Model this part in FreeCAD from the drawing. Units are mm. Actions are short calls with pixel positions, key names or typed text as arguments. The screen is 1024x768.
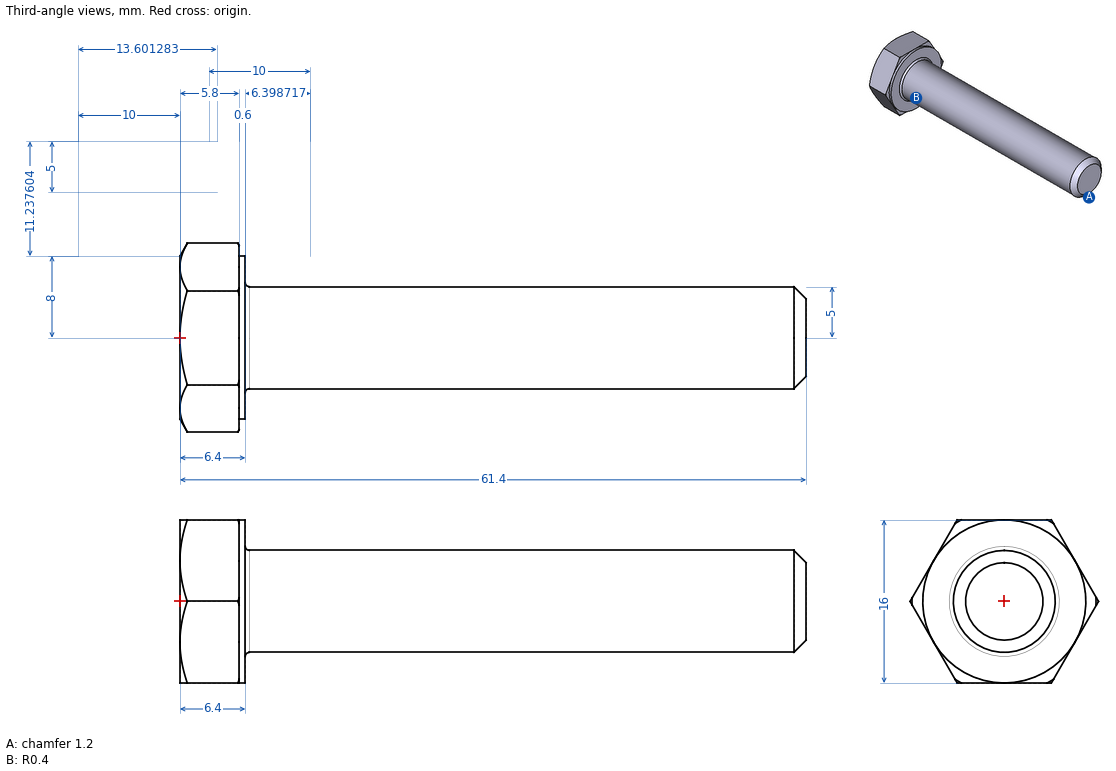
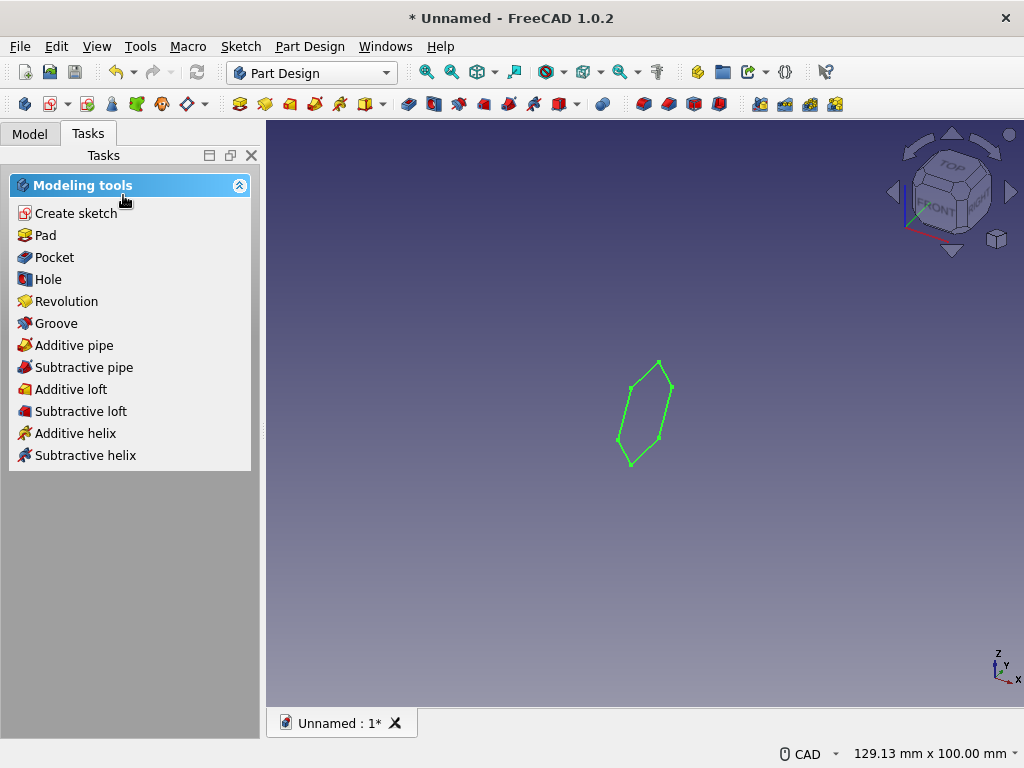
click(240, 104)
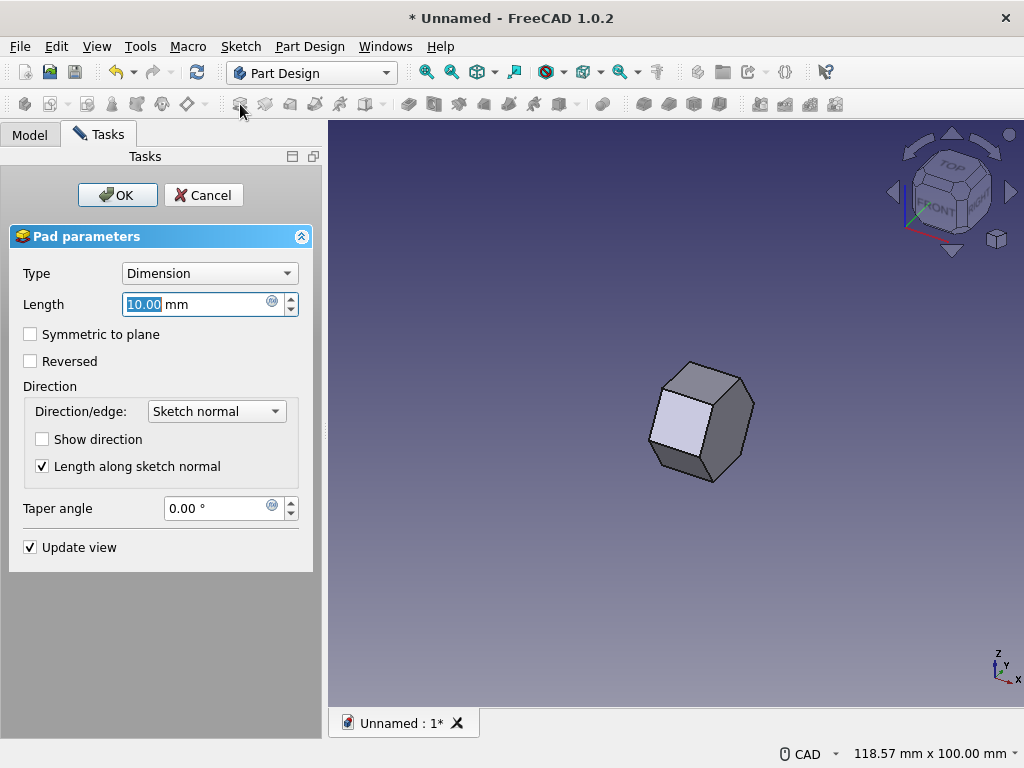
text(6.4)
key(Tab)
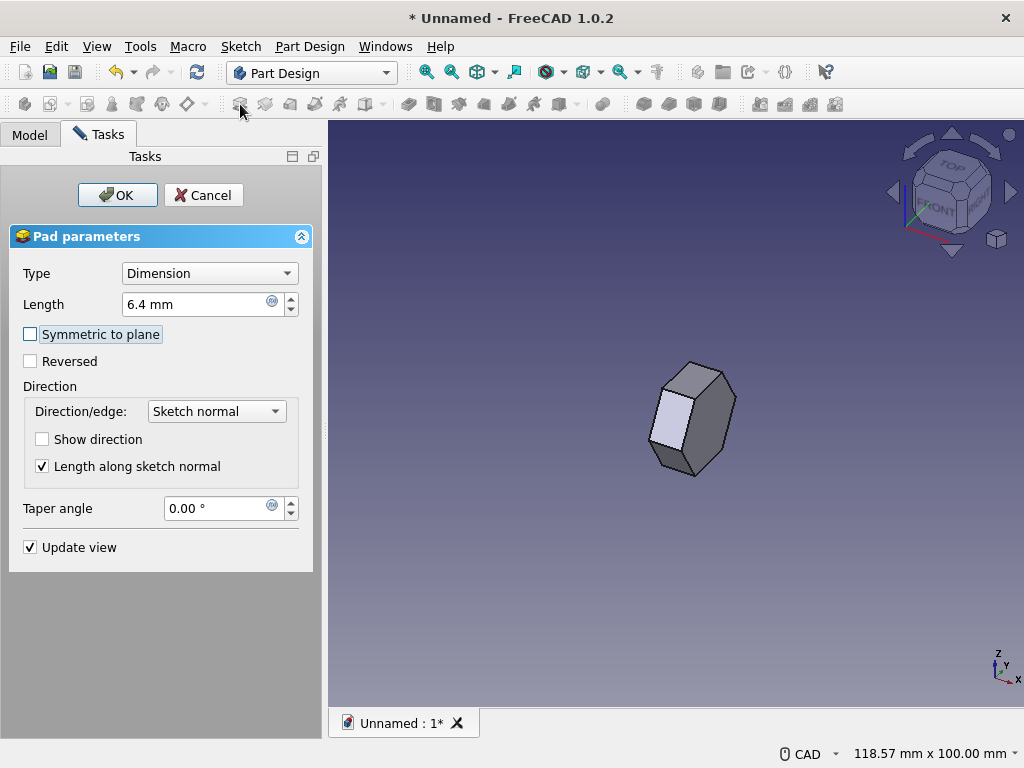
click(118, 195)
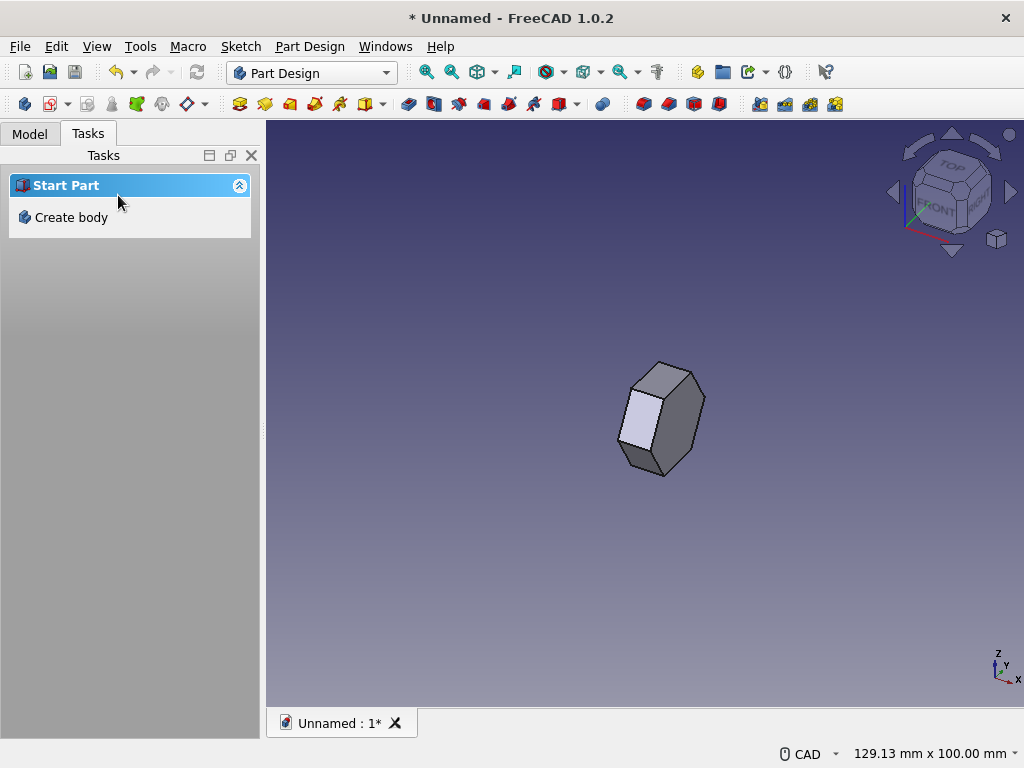
click(427, 72)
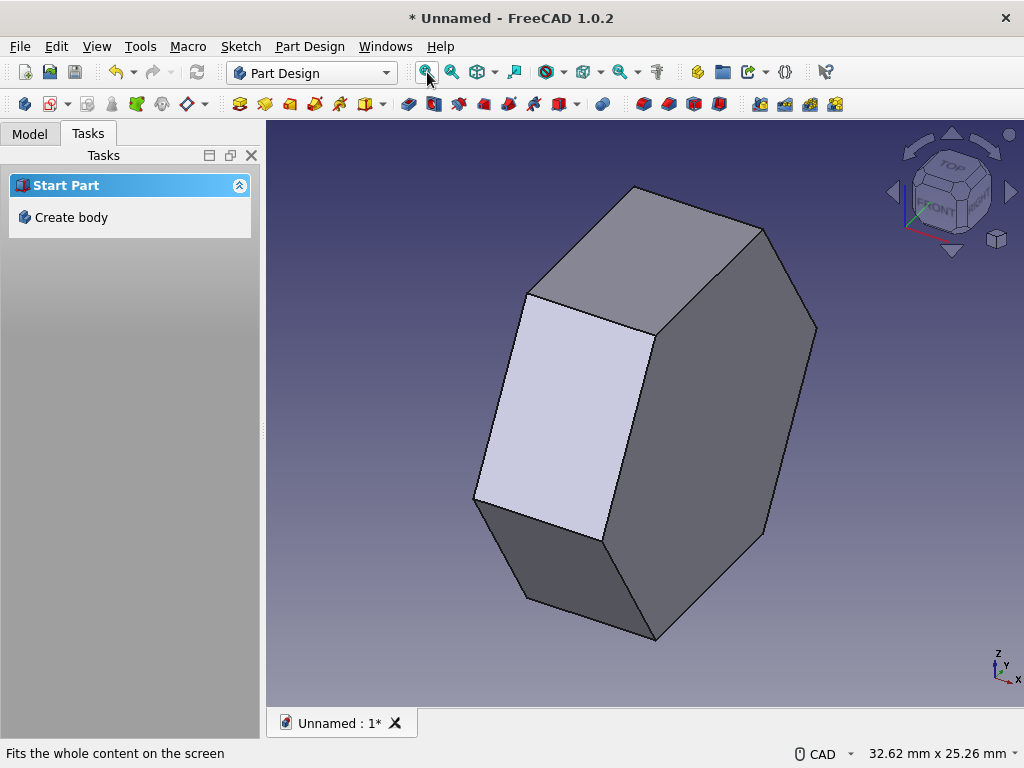
click(50, 104)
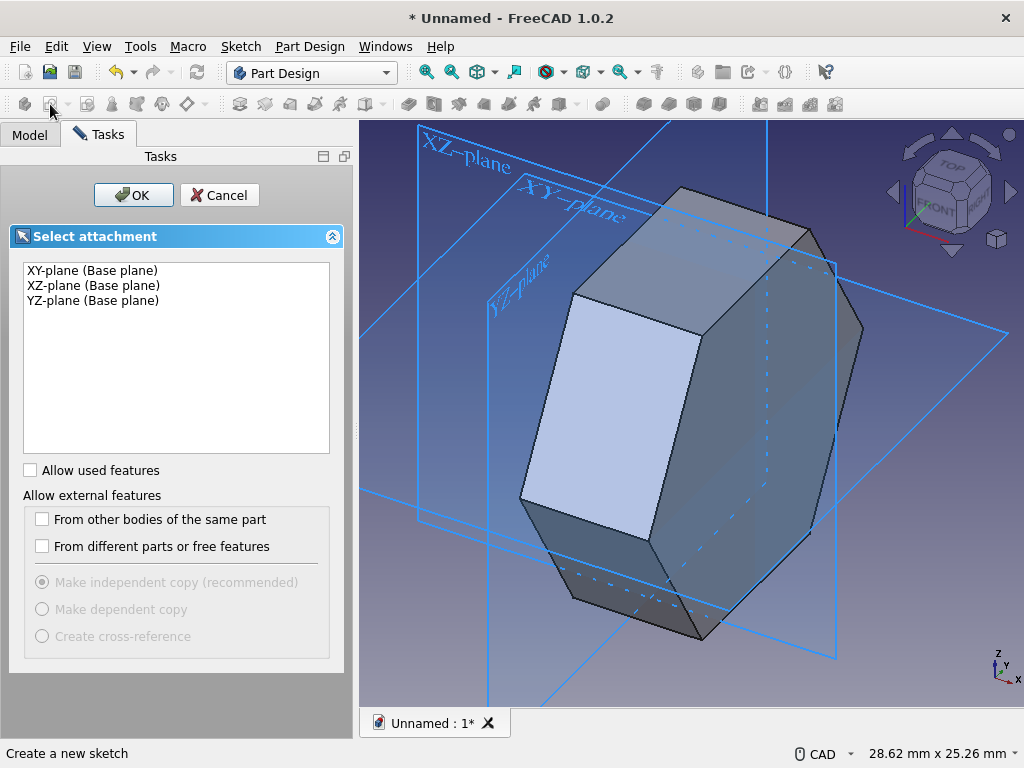
click(84, 270)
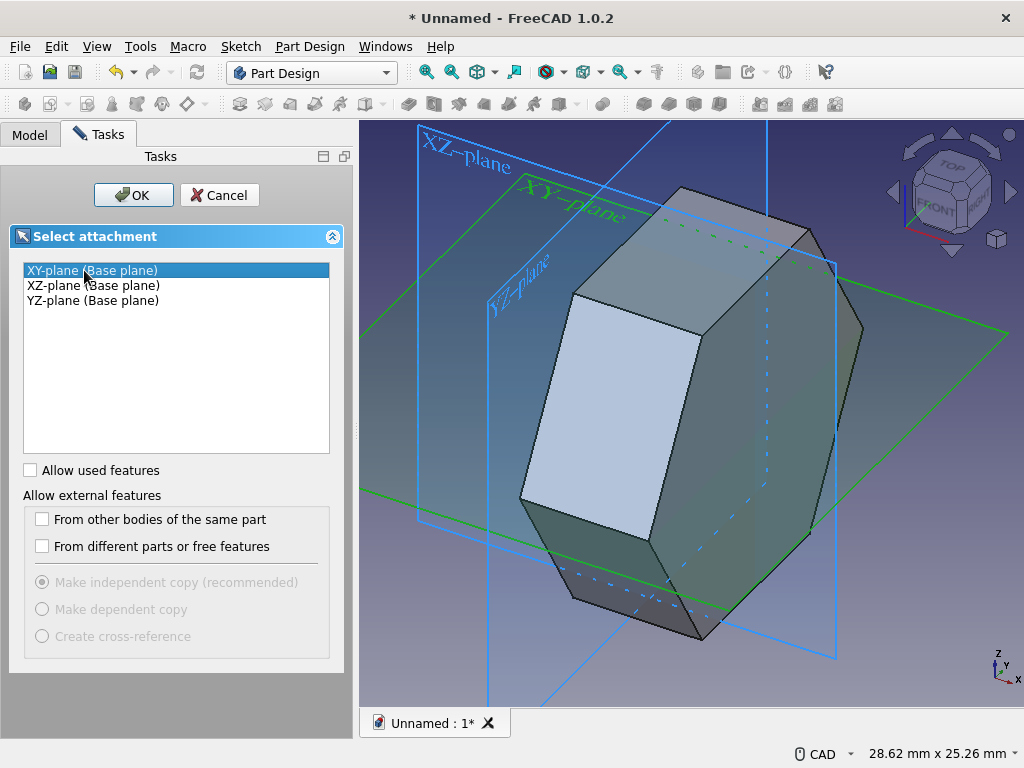
click(134, 195)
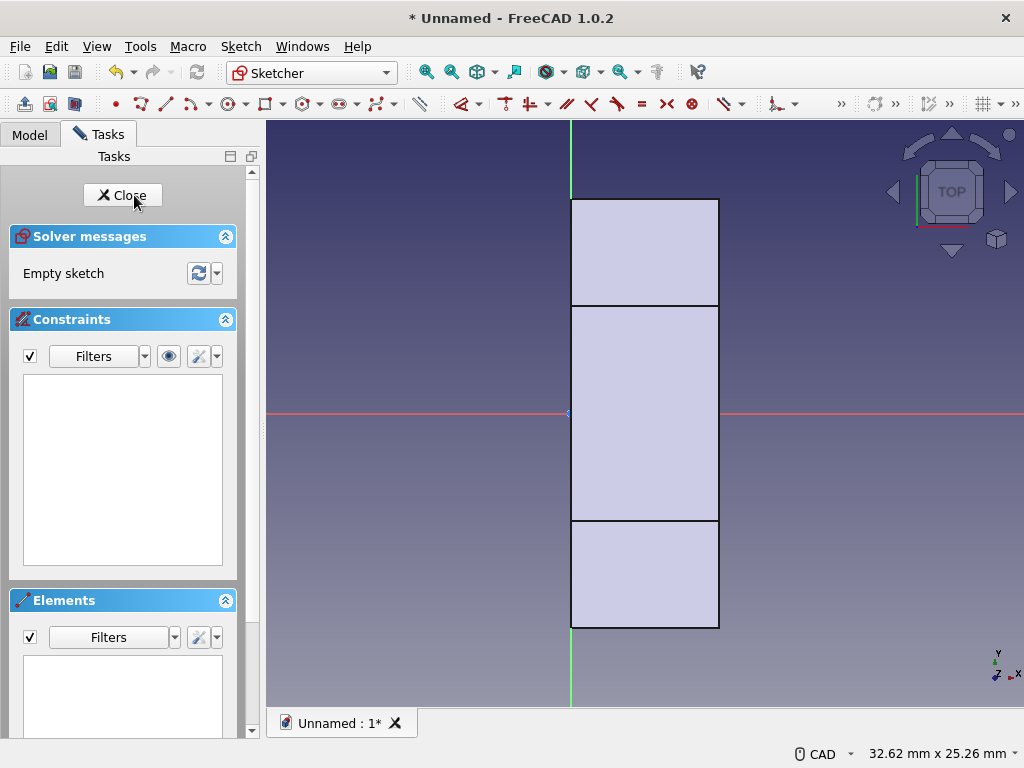
click(75, 104)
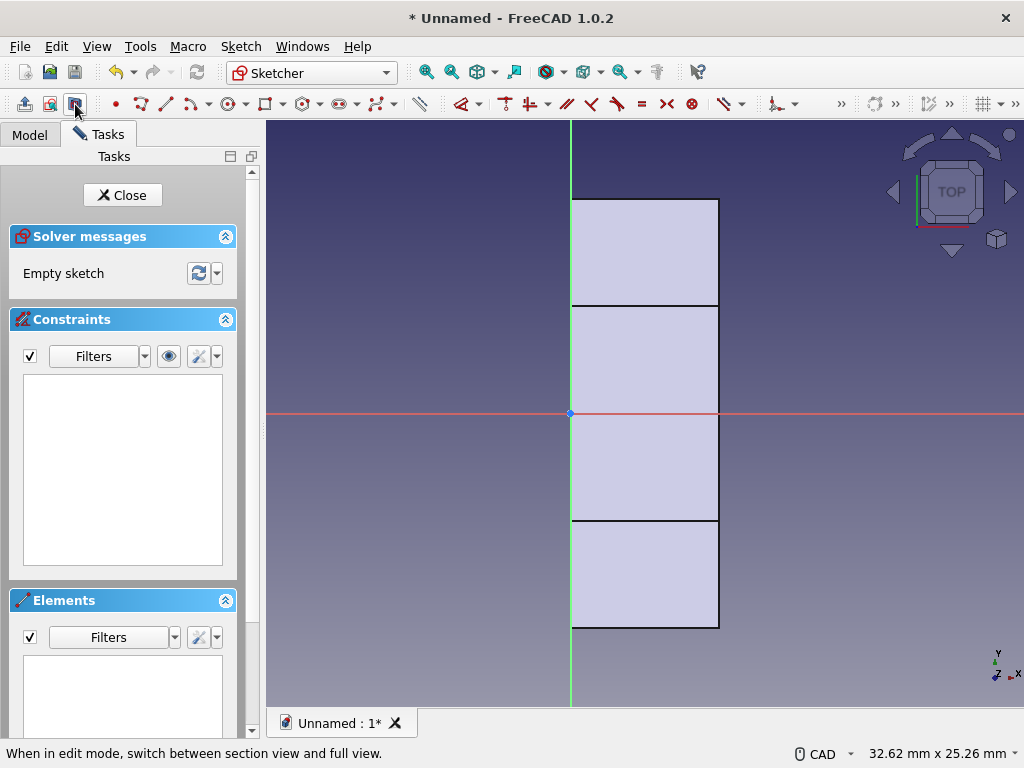
scroll(294, 439, down, 6)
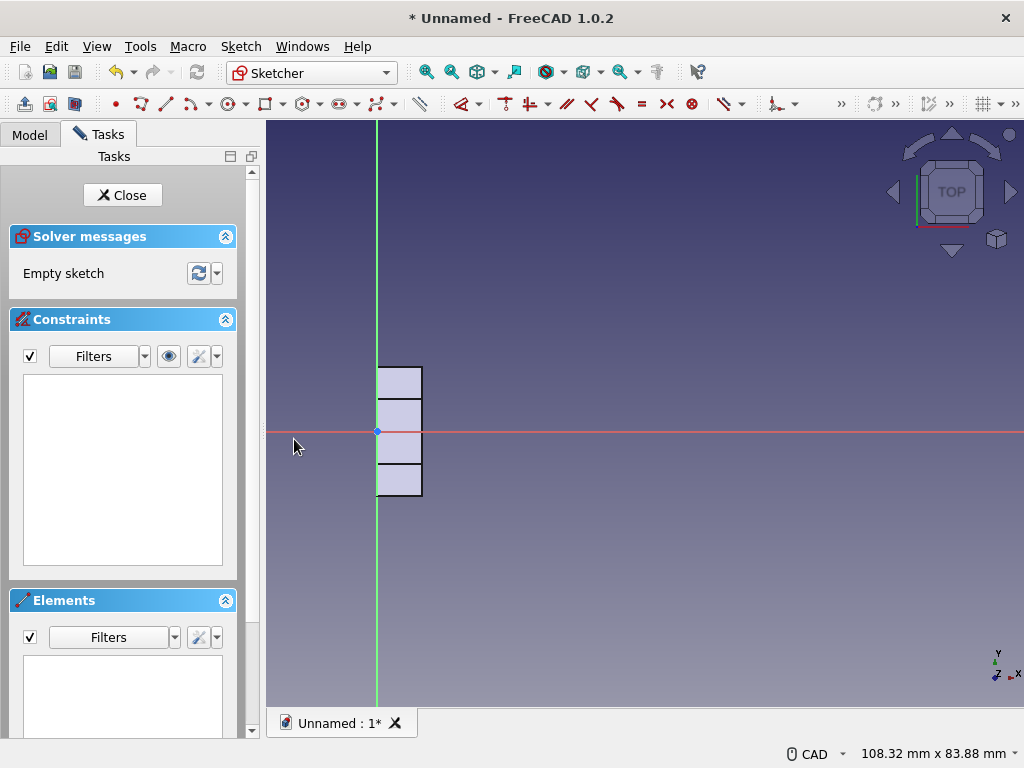
click(264, 104)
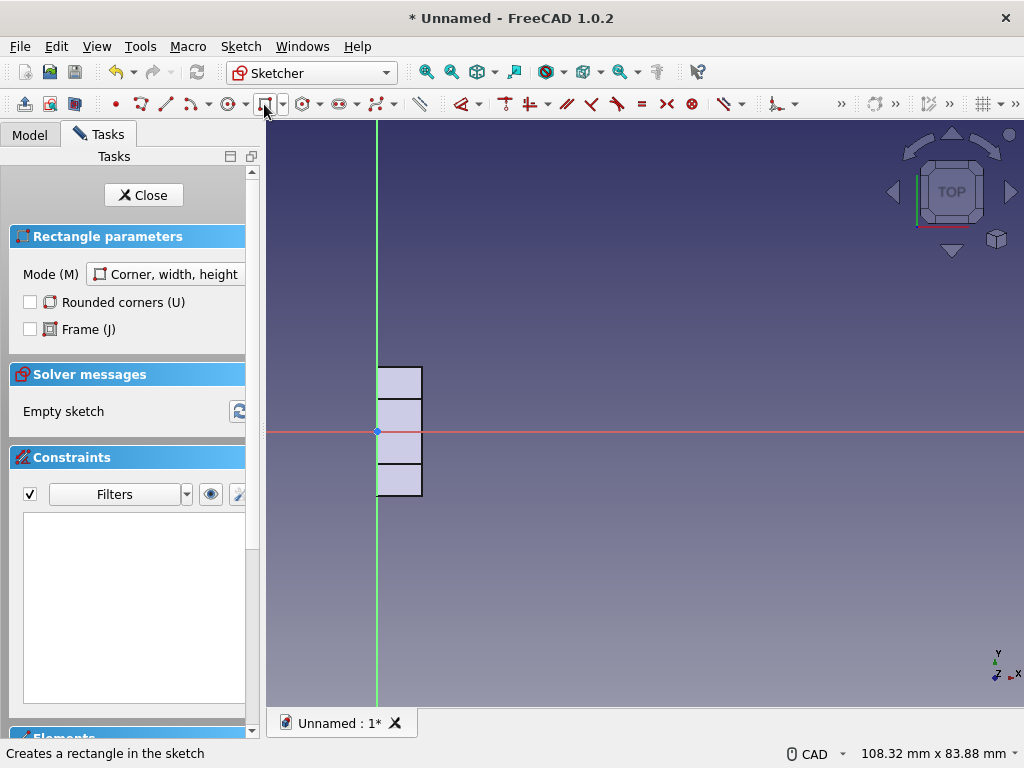
click(377, 432)
move(807, 397)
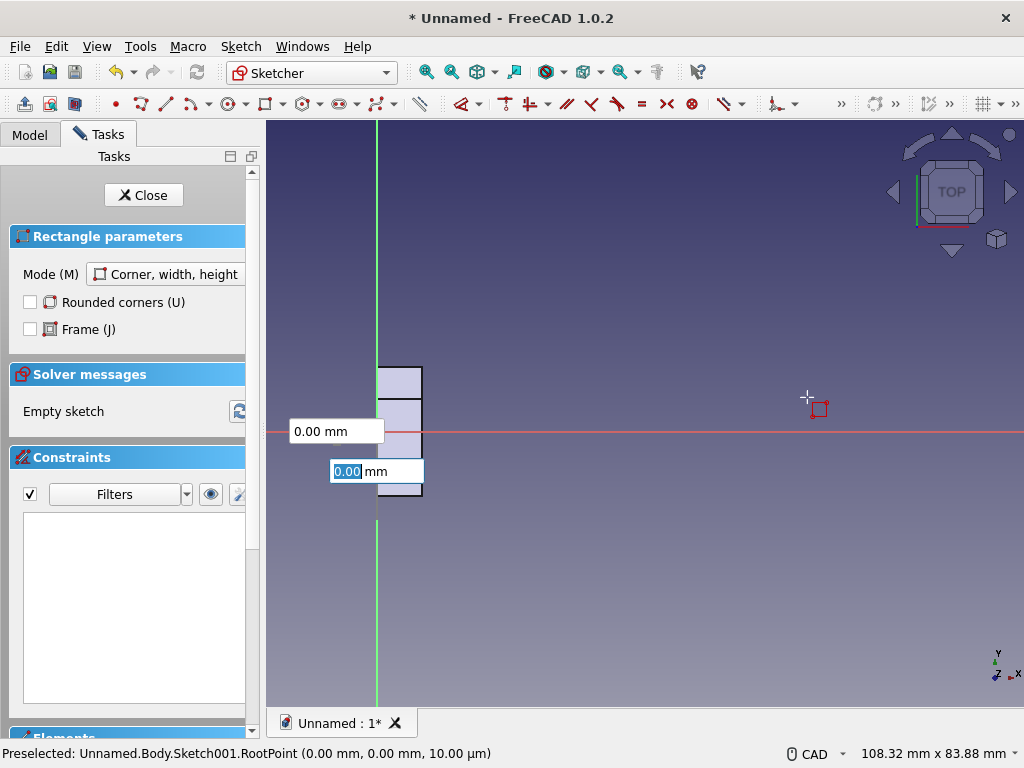
text(61.4)
key(Tab)
text(5)
key(Return)
key(Escape)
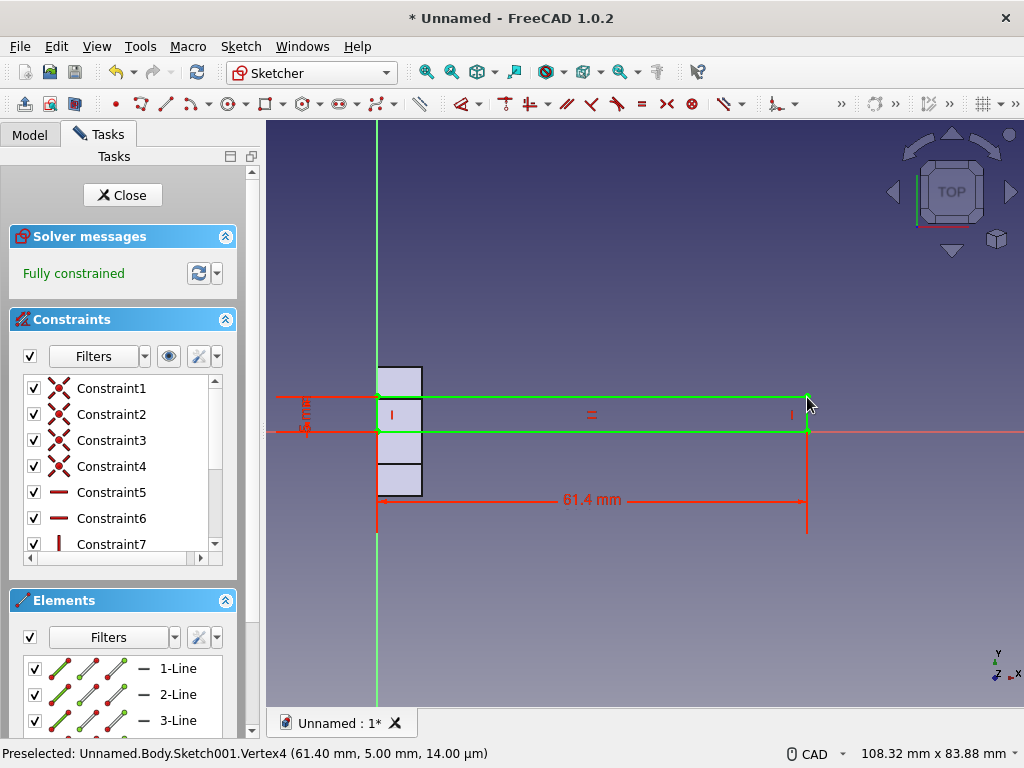
click(123, 195)